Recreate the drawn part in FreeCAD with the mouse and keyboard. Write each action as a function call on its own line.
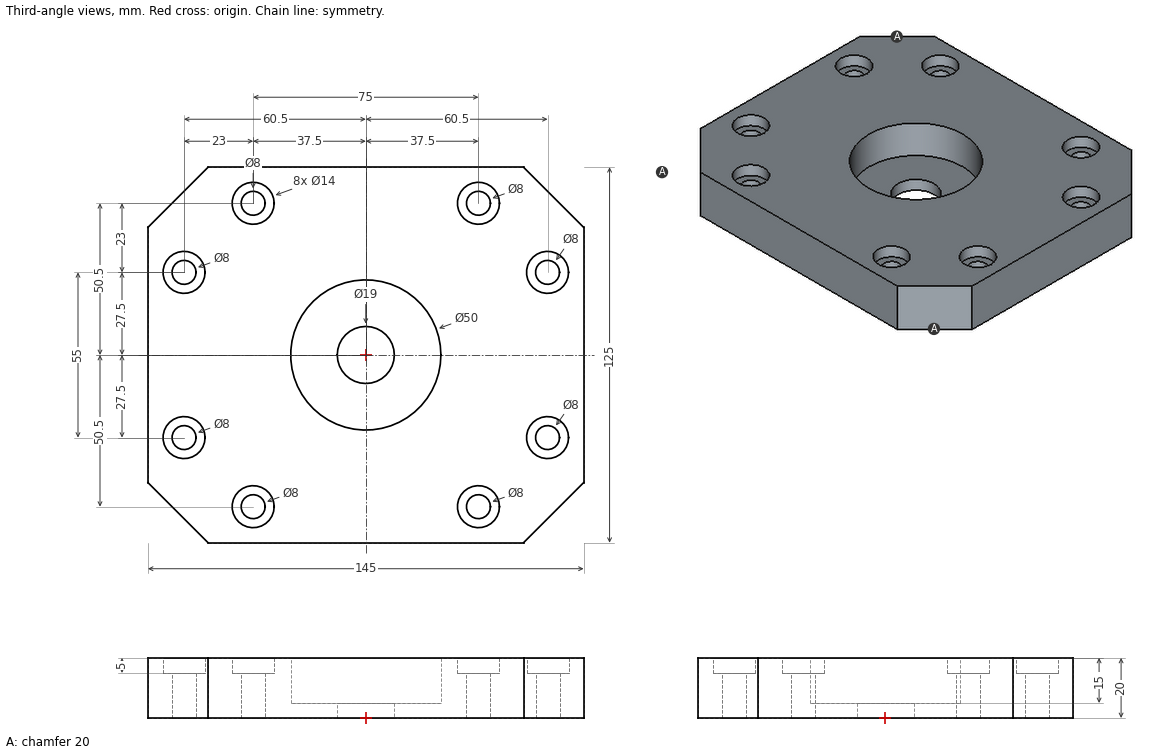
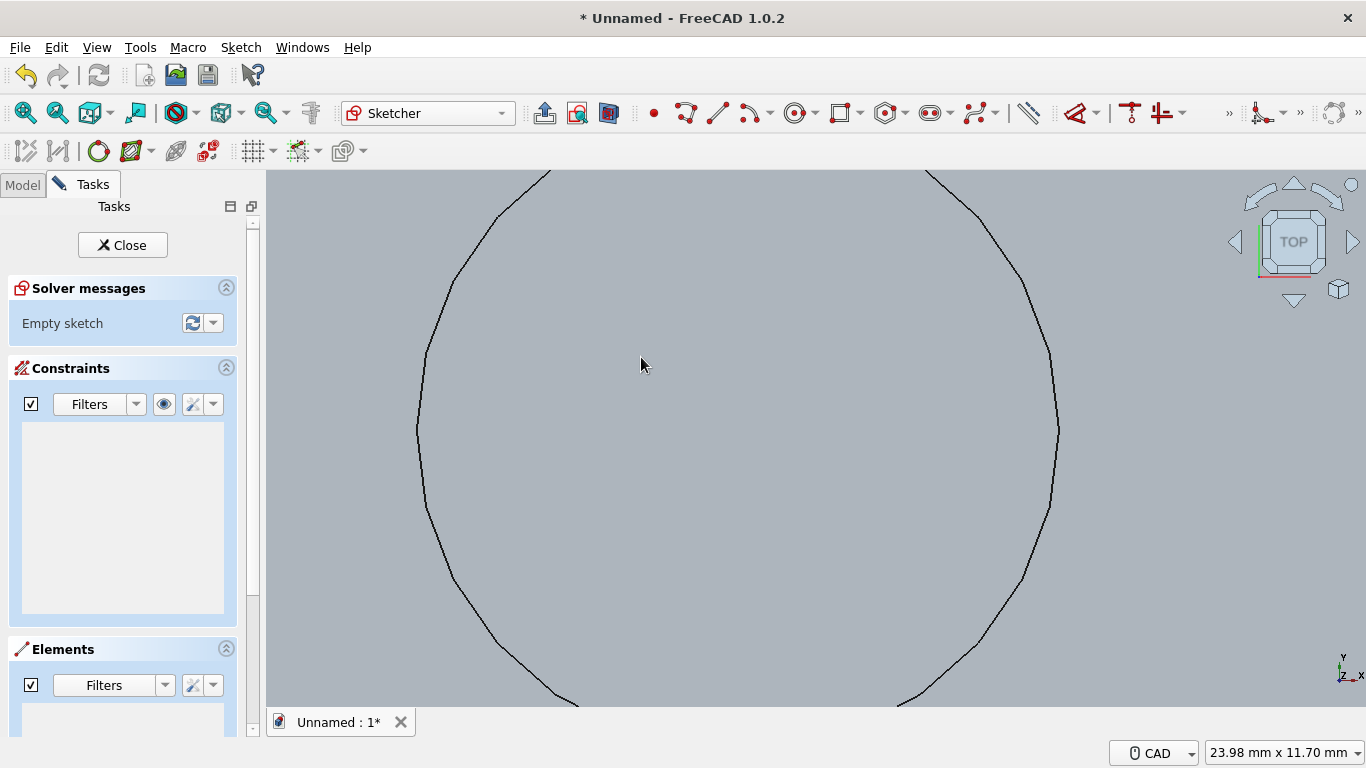
click(796, 114)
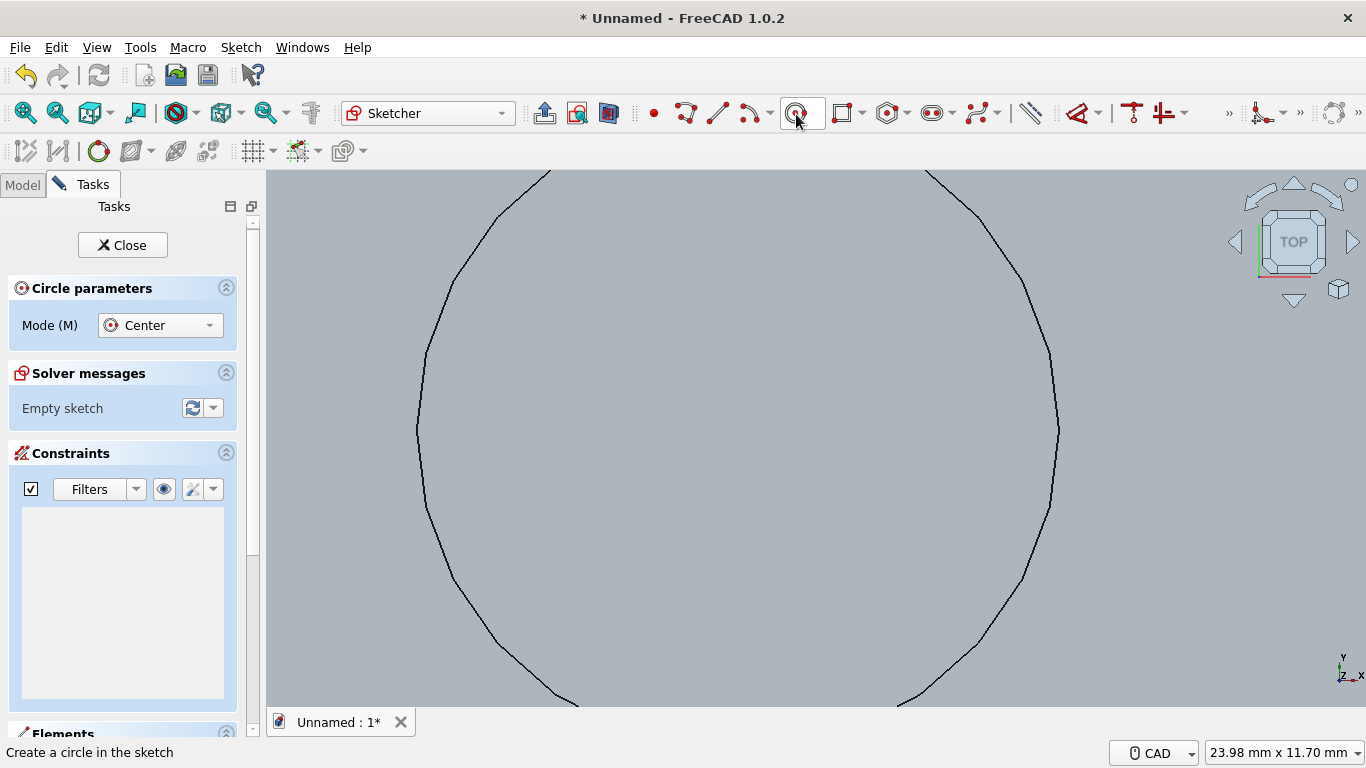
click(738, 430)
click(868, 300)
key(Escape)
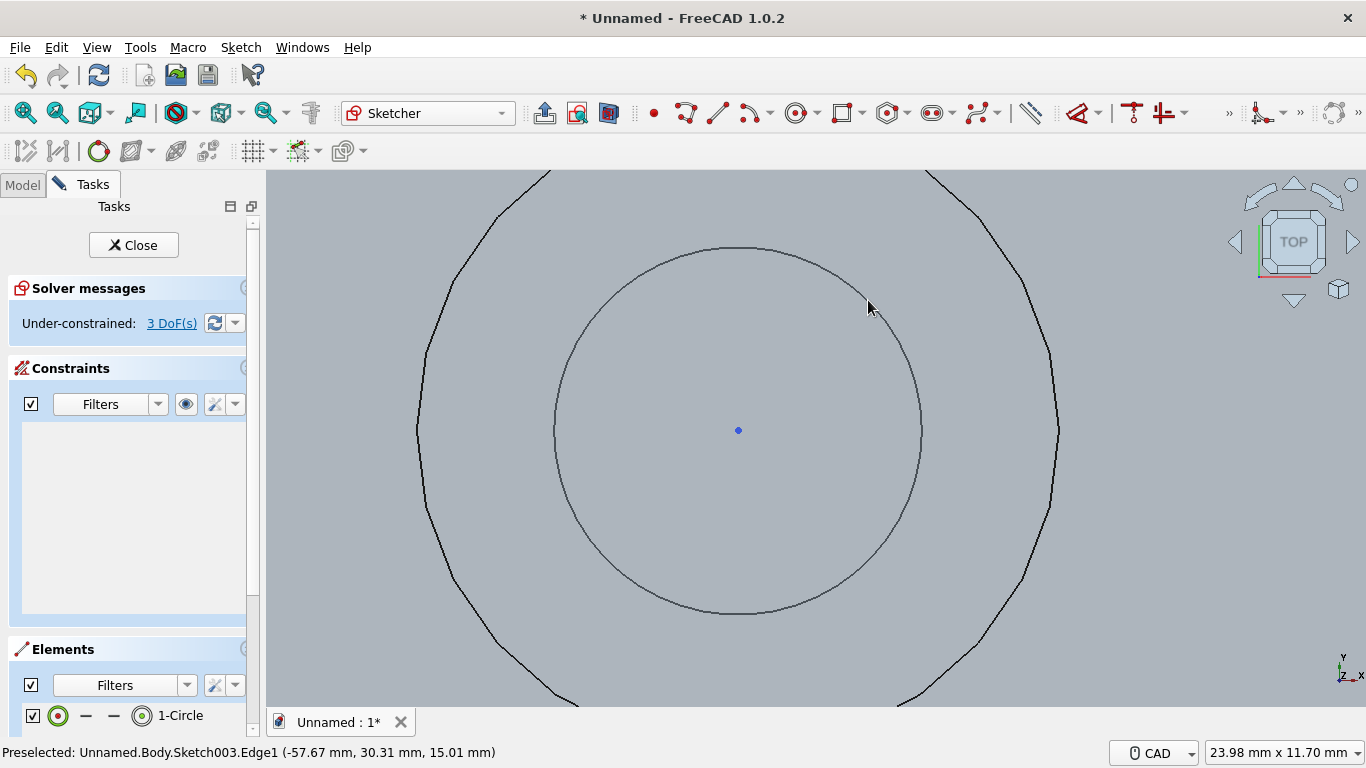
click(1078, 114)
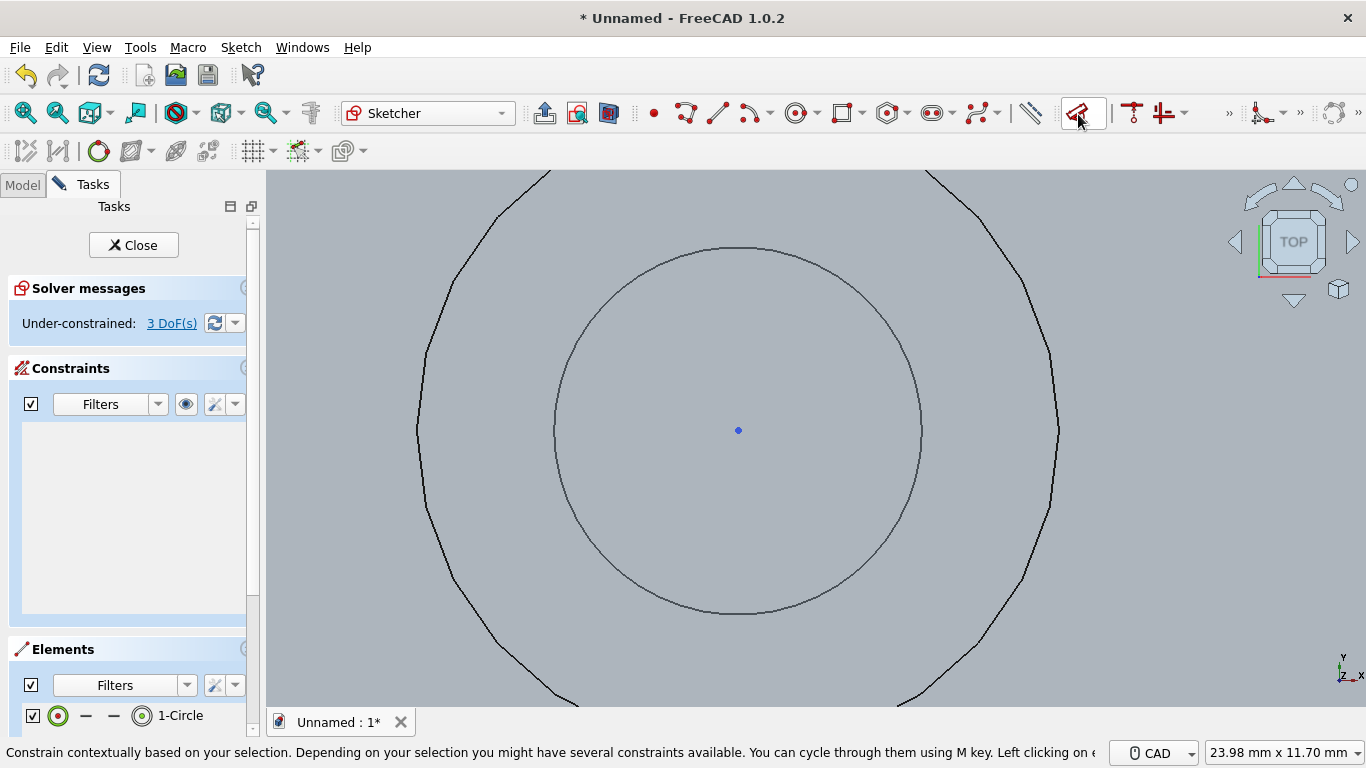
click(868, 301)
click(891, 278)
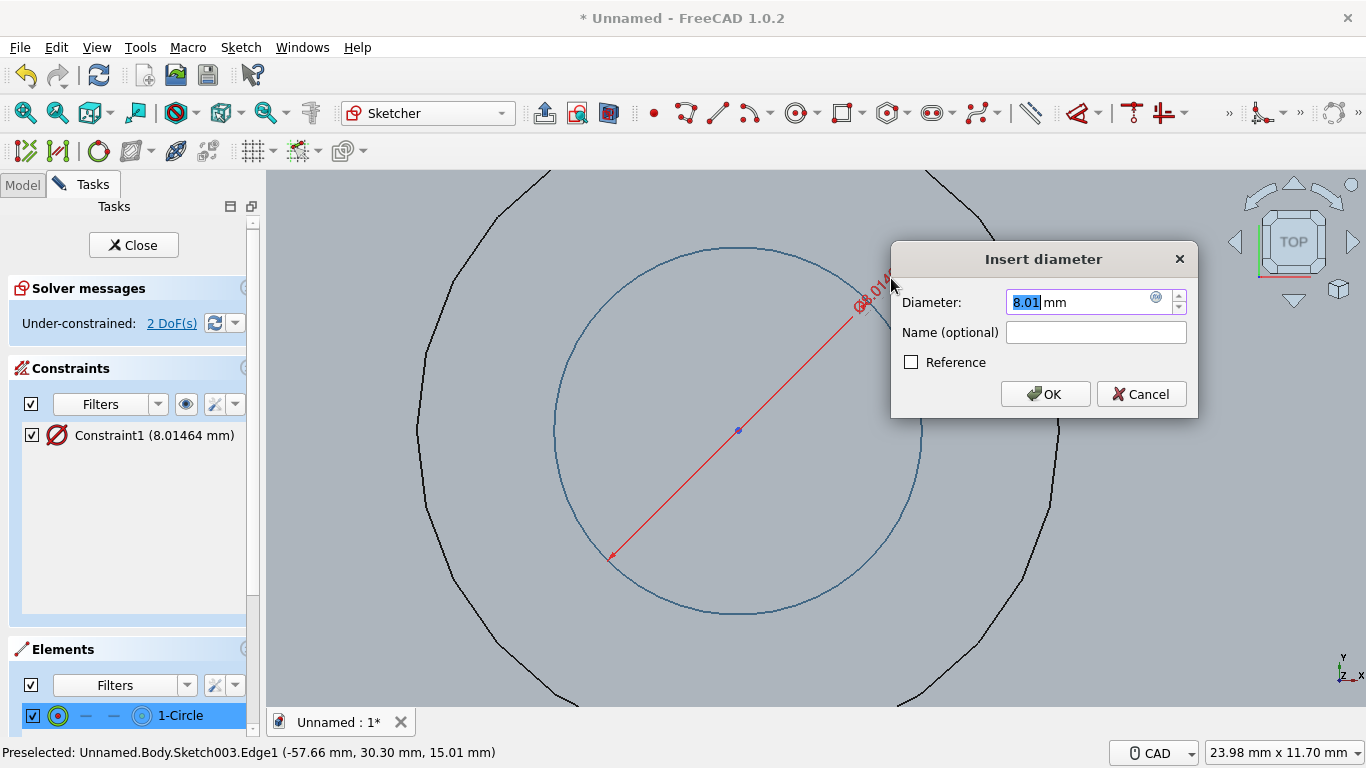
text(8)
key(Return)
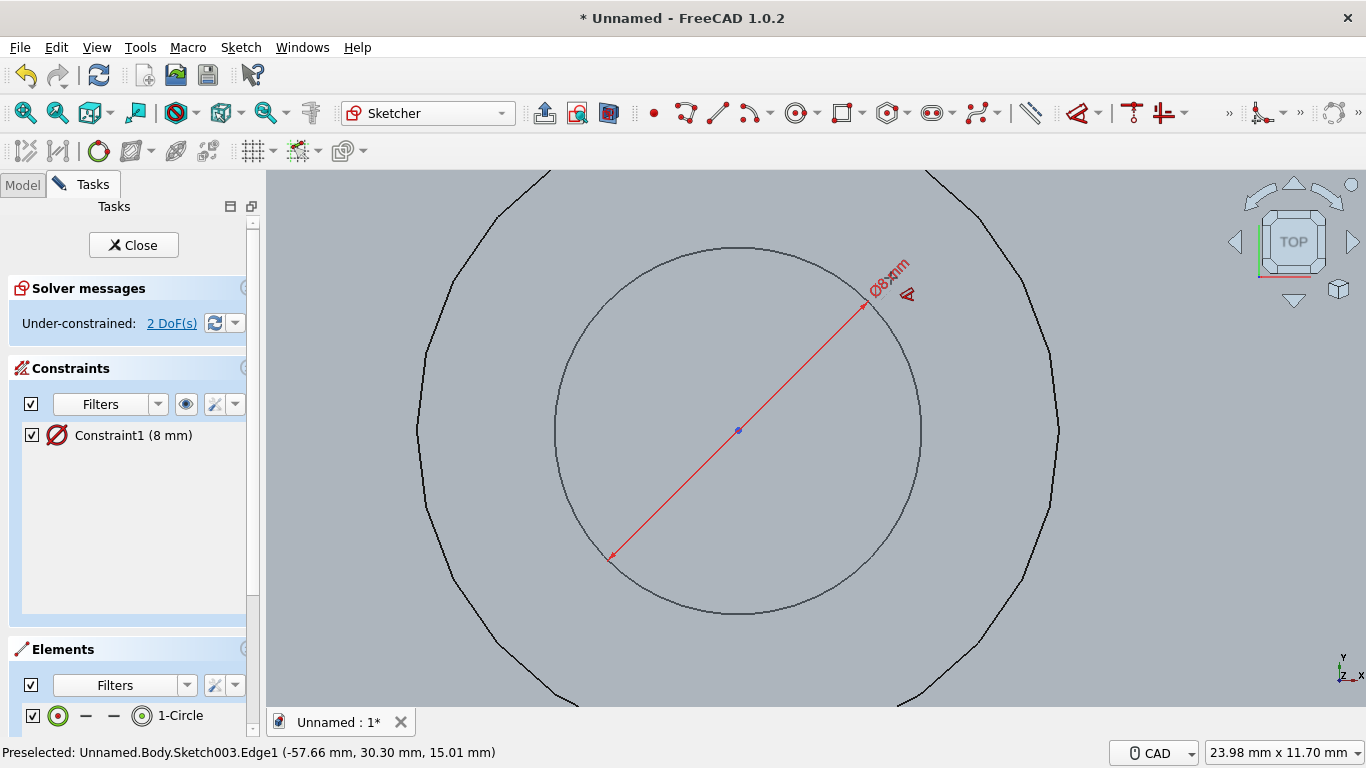
click(738, 431)
click(970, 397)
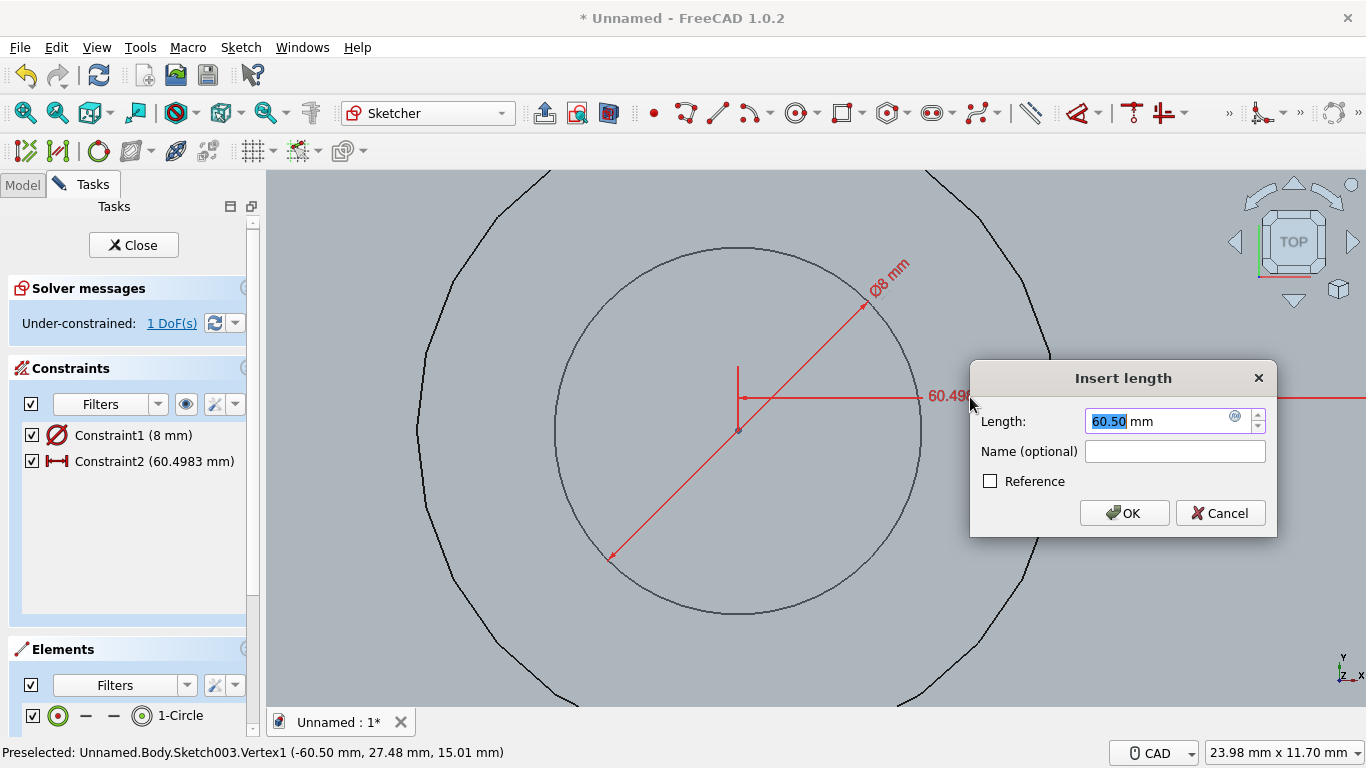
text(60.5)
key(Return)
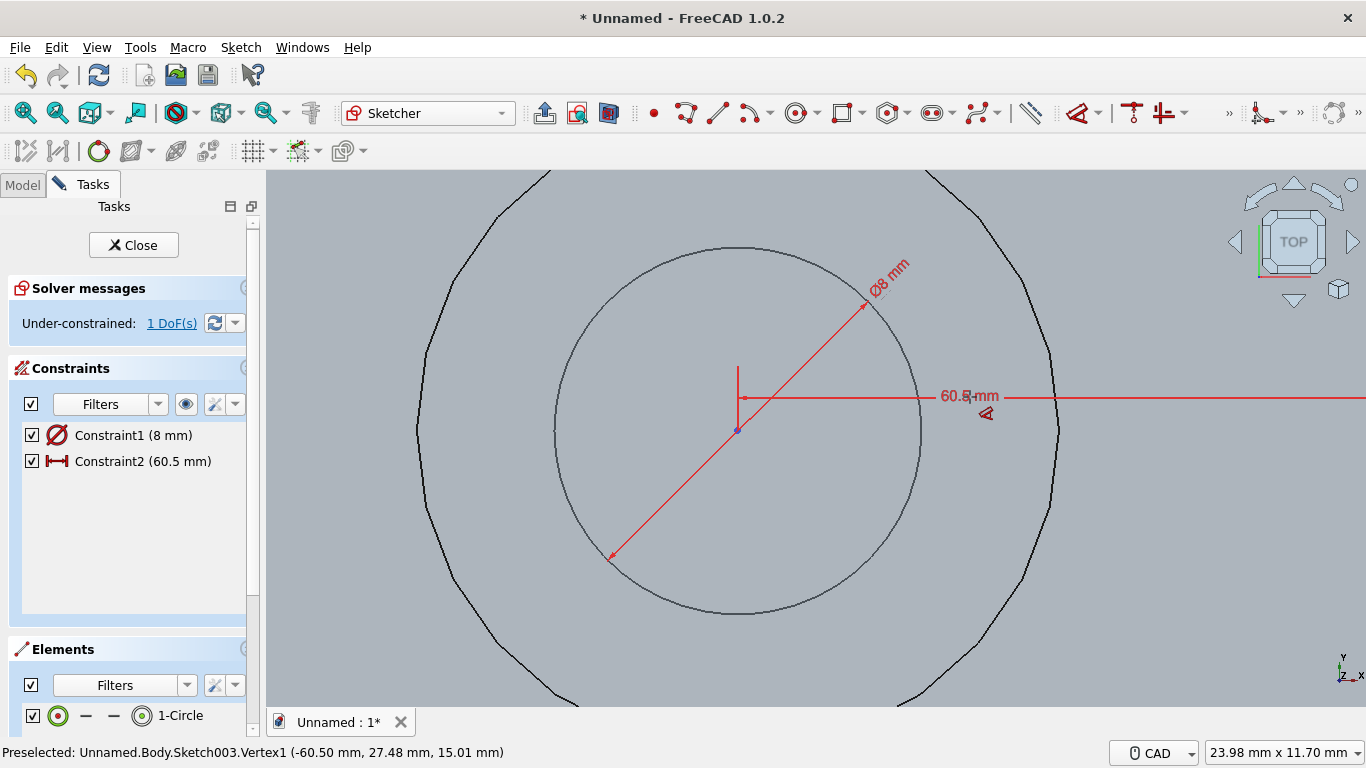
click(738, 431)
click(704, 555)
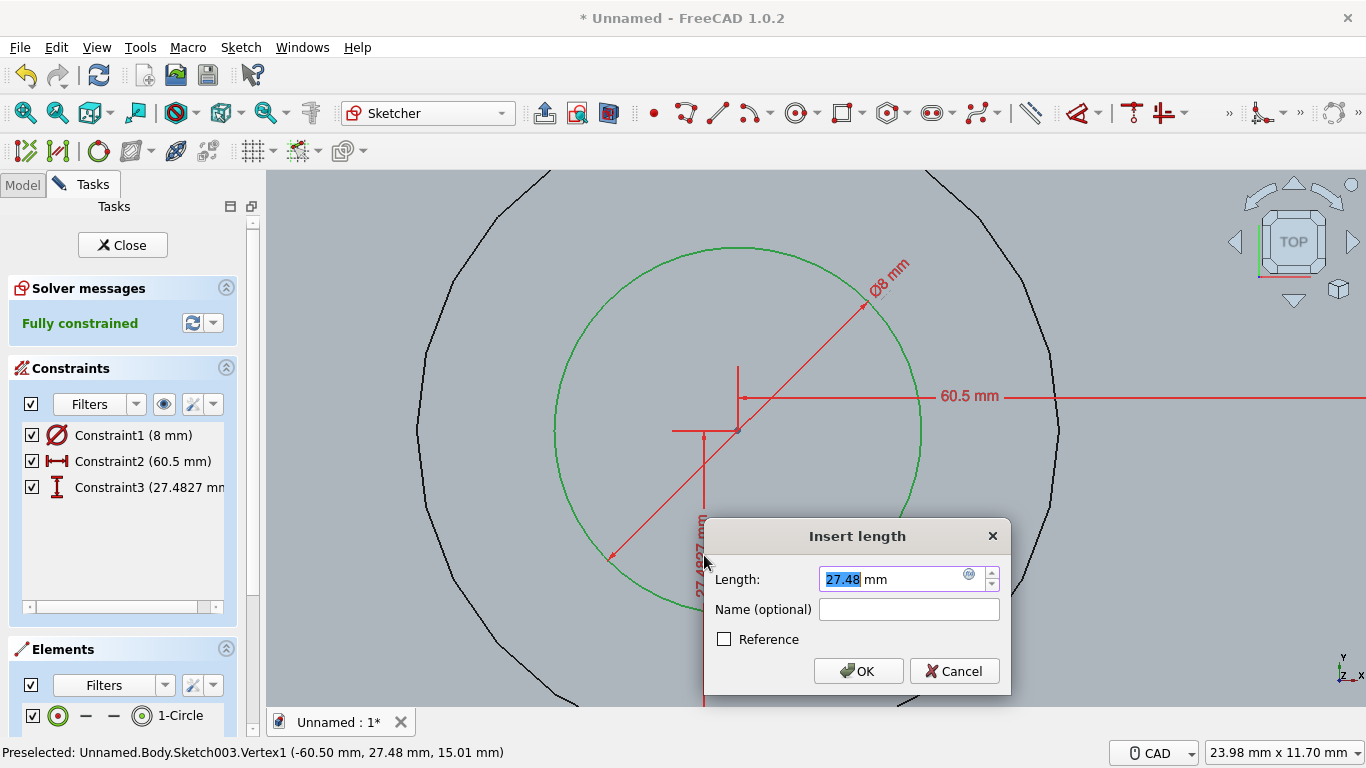
text(27.5)
key(Return)
key(Escape)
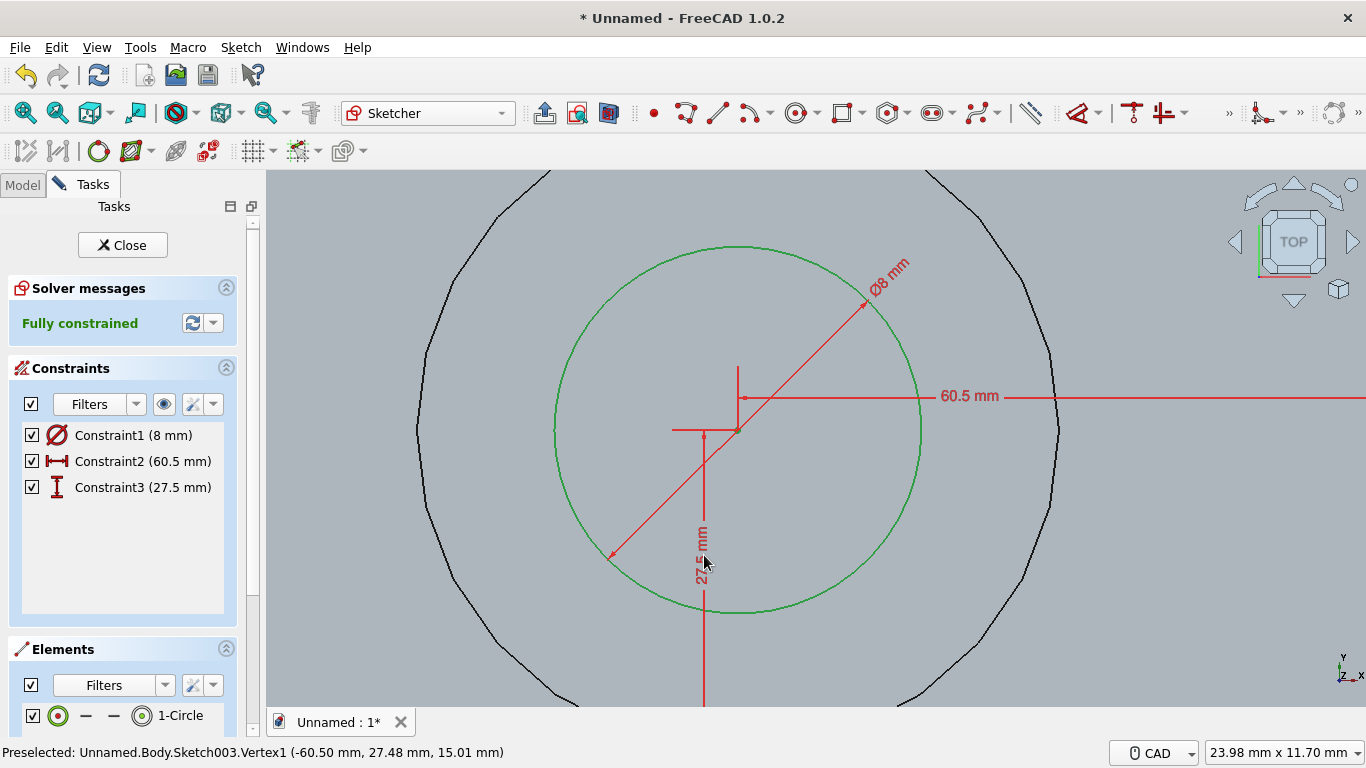
click(123, 245)